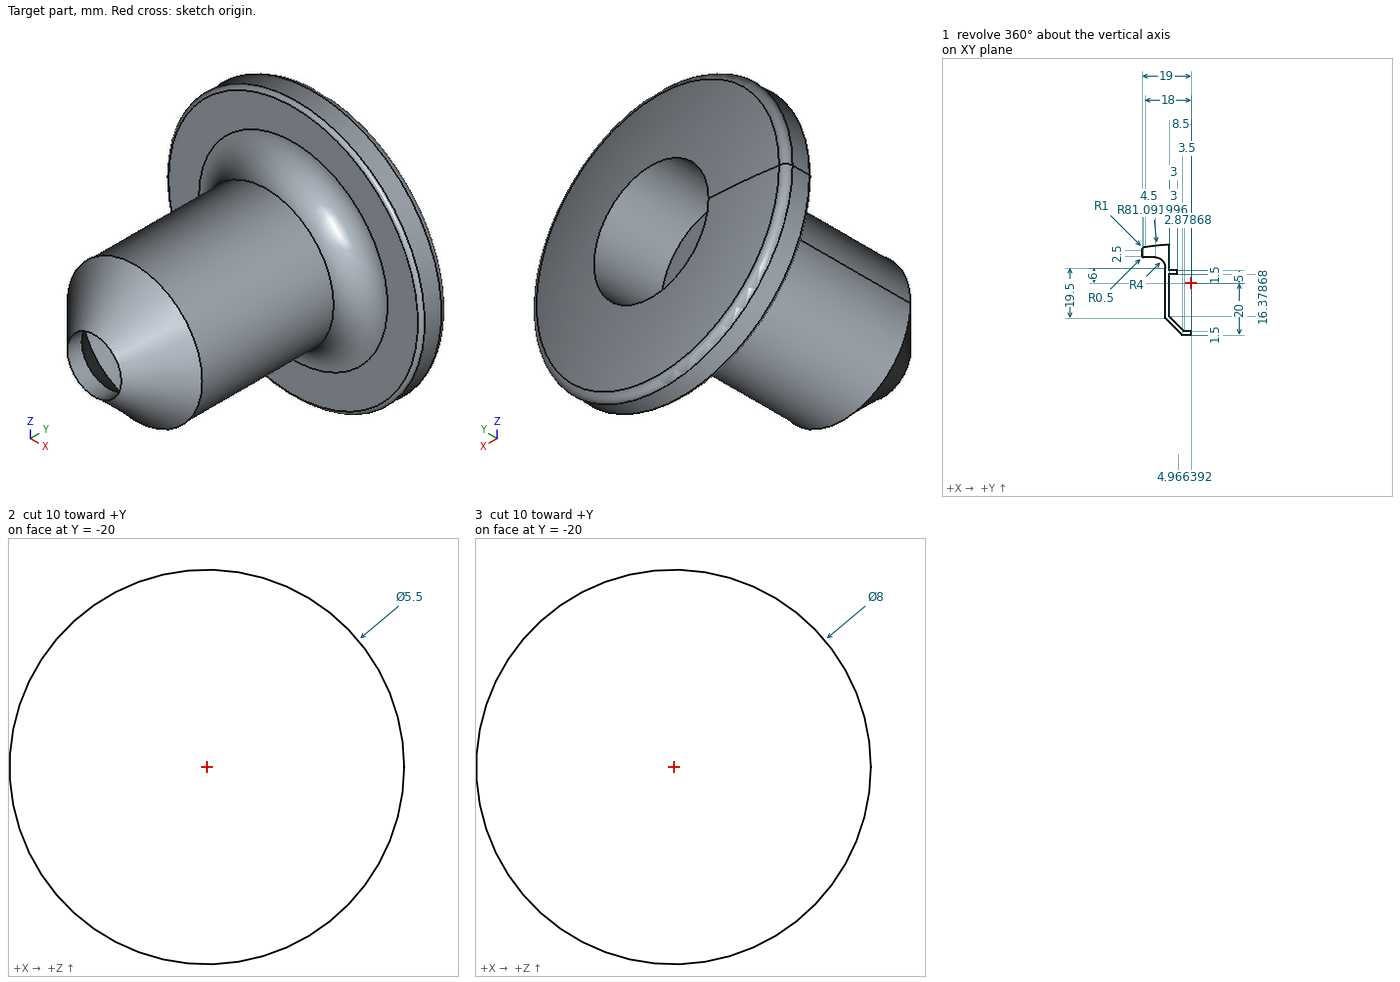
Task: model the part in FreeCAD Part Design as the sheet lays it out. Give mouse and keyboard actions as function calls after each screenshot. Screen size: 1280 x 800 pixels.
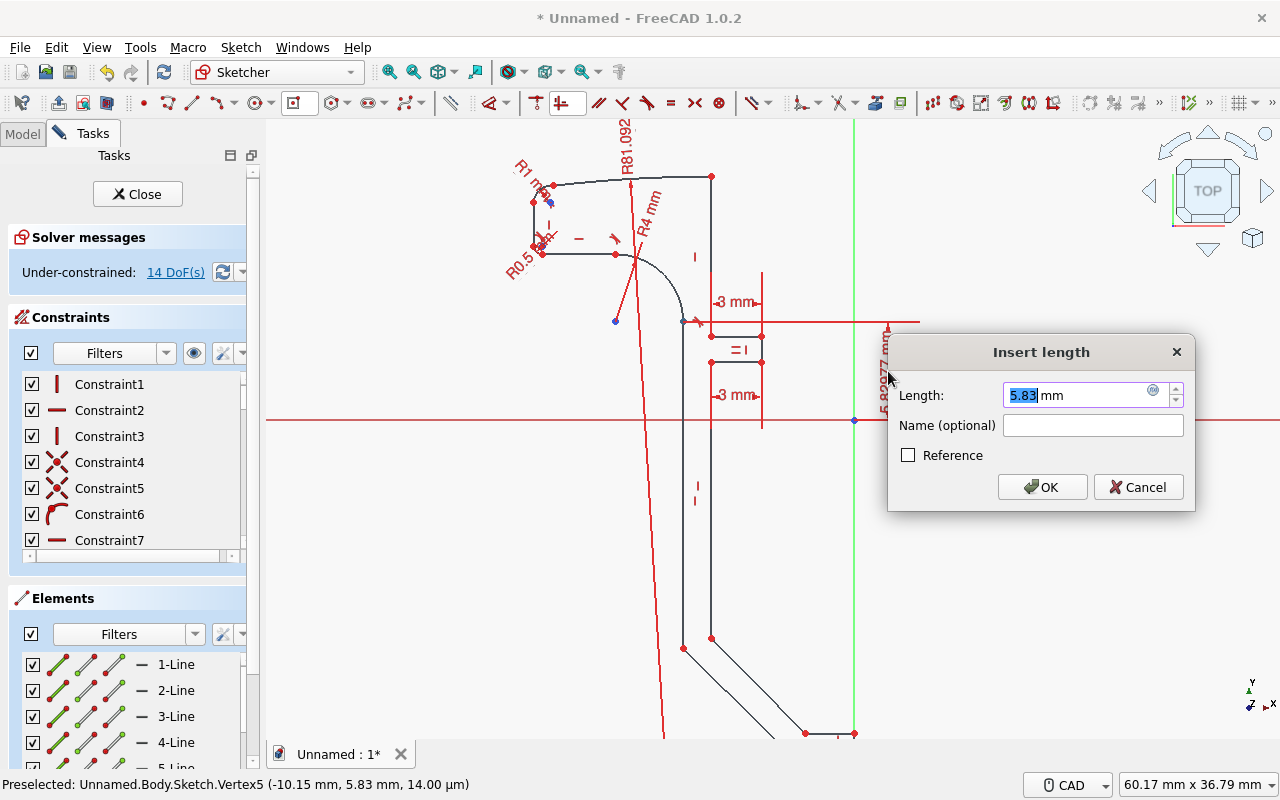
text(6)
key(Return)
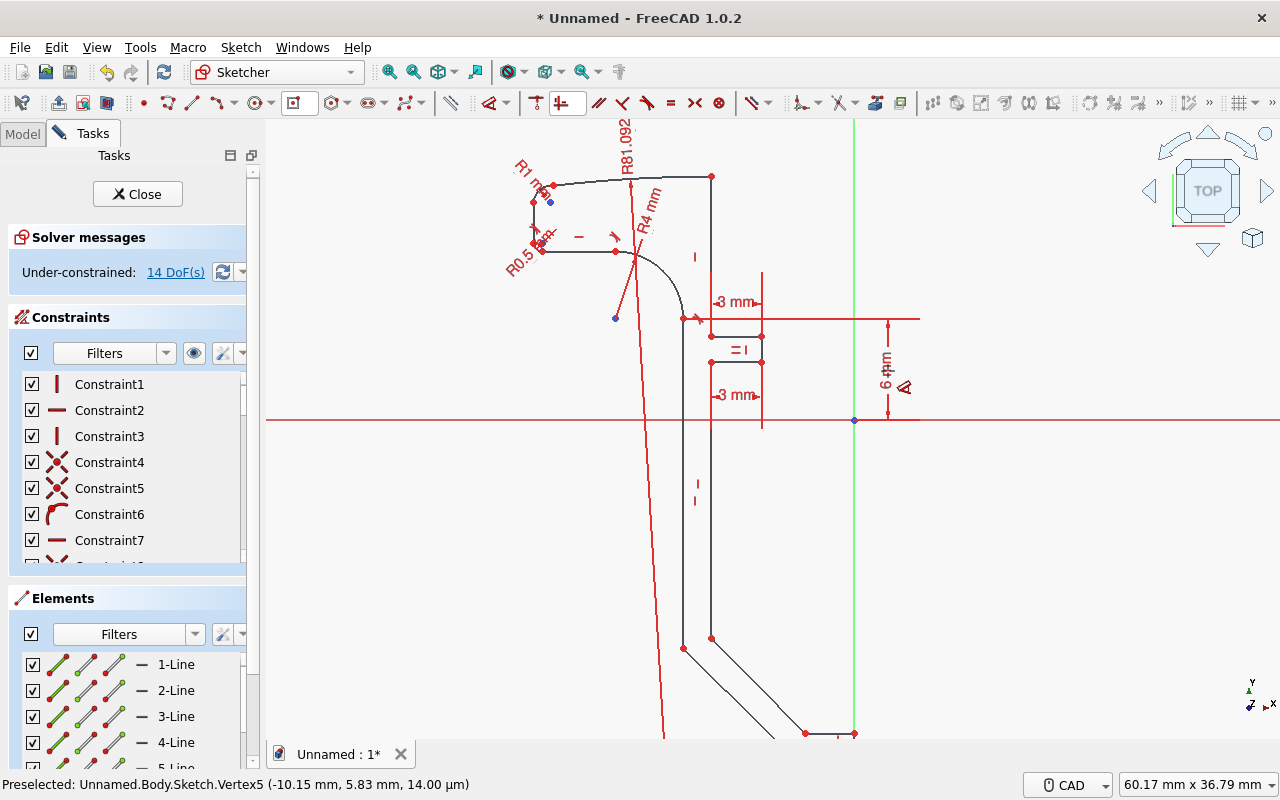
click(762, 337)
click(888, 398)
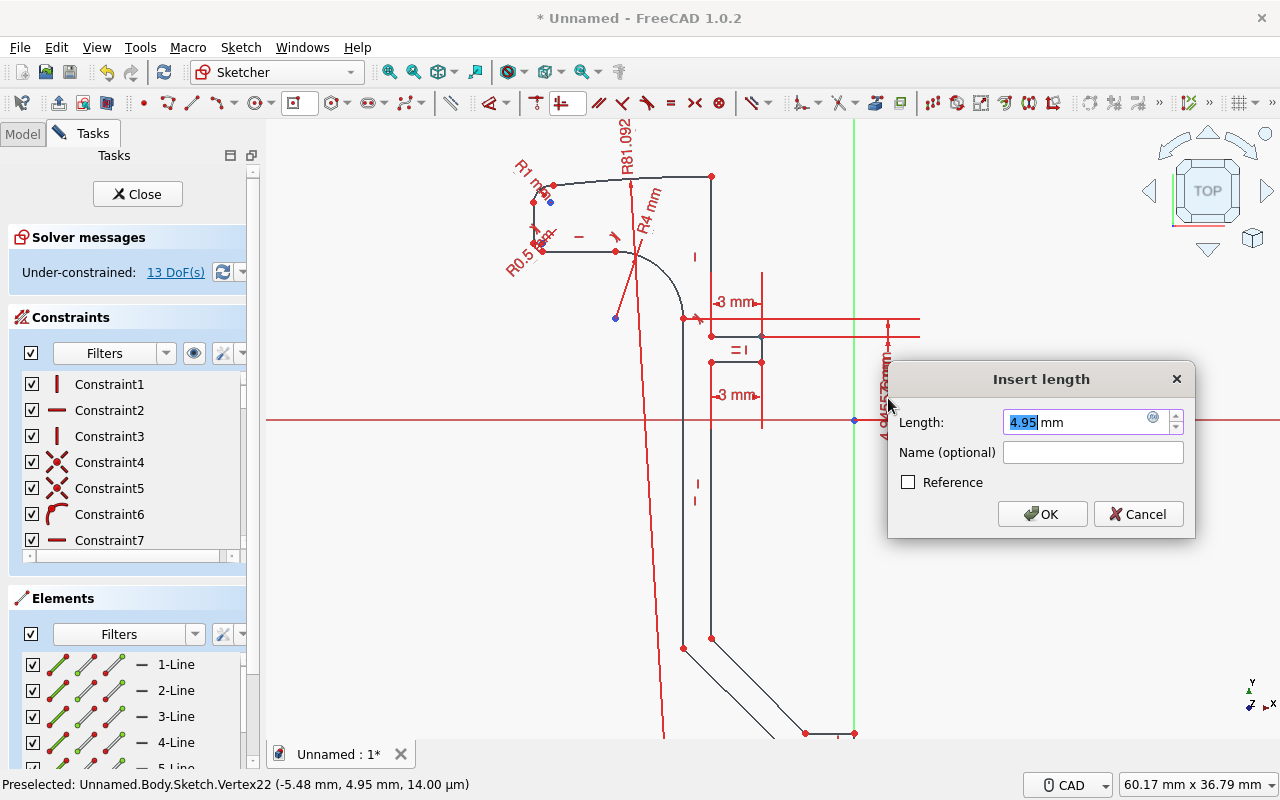
text(5)
key(Return)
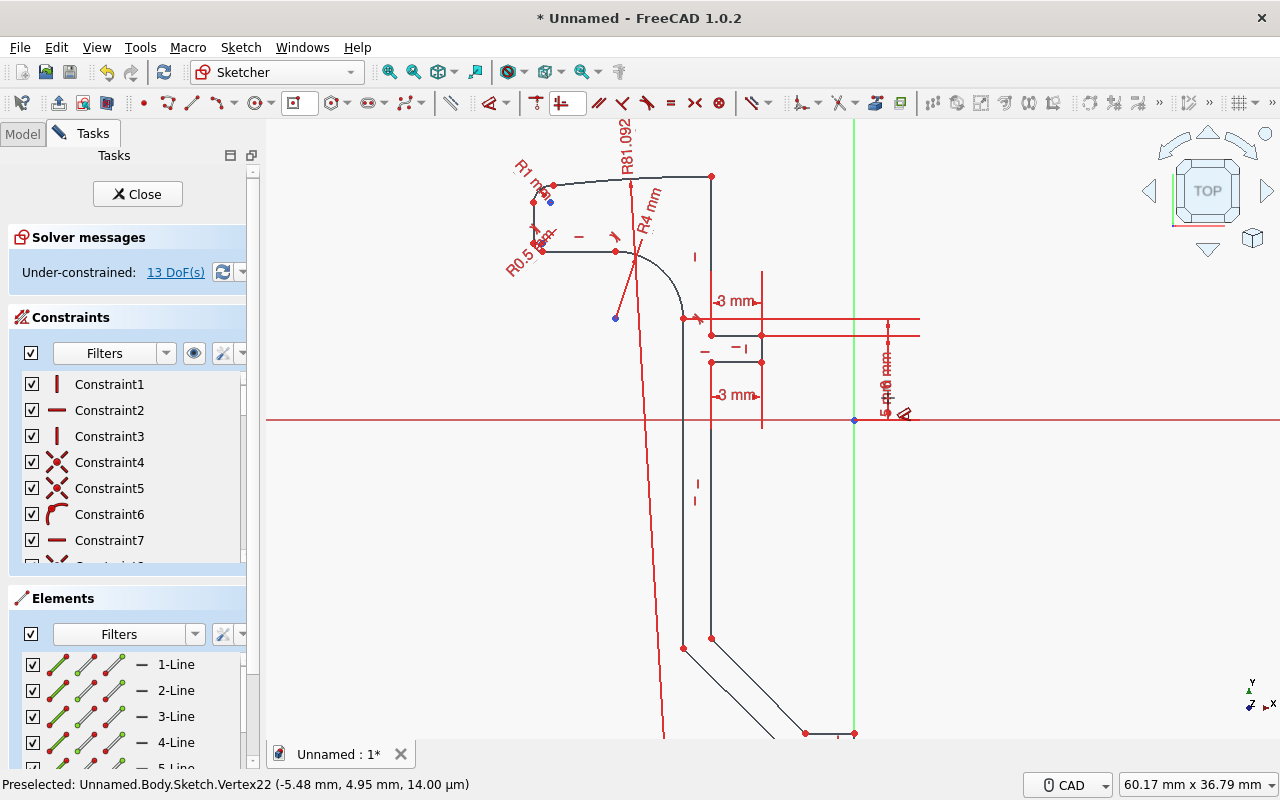
click(534, 215)
click(500, 223)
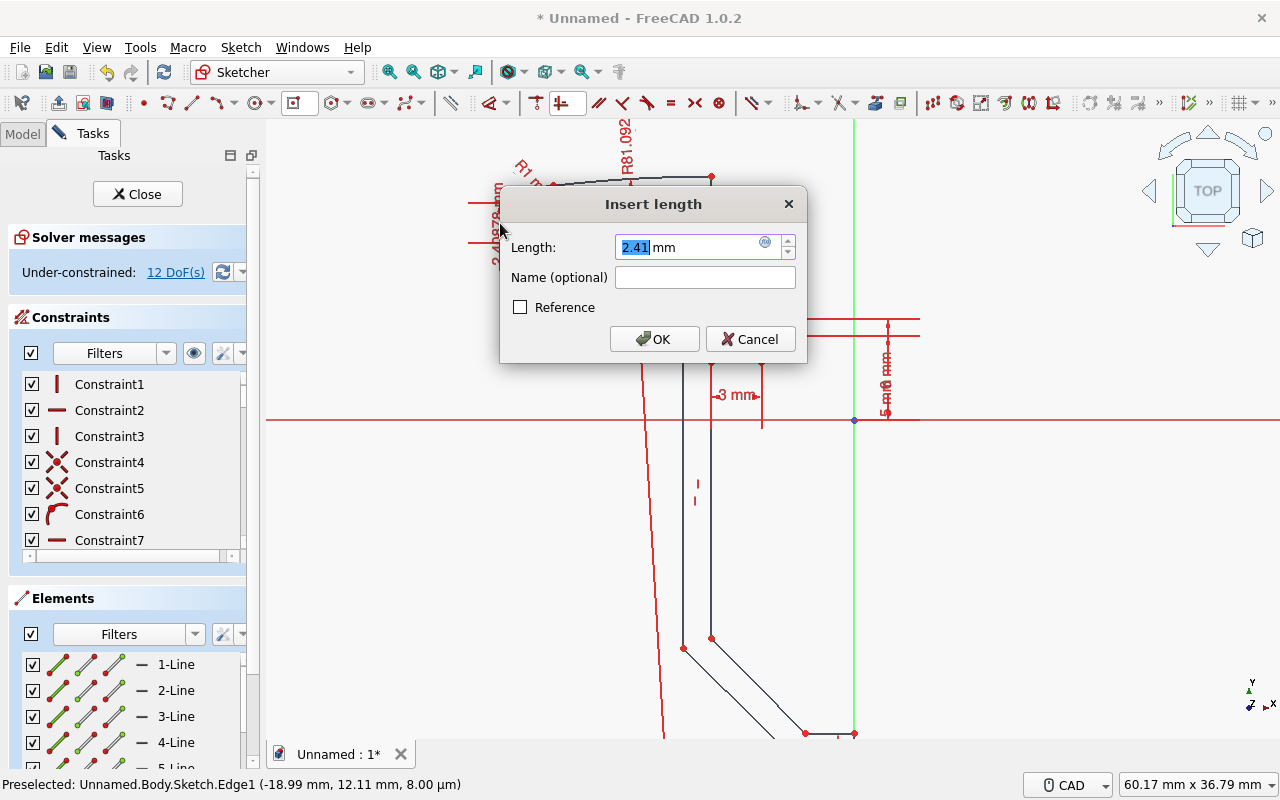
text(2.5)
key(Return)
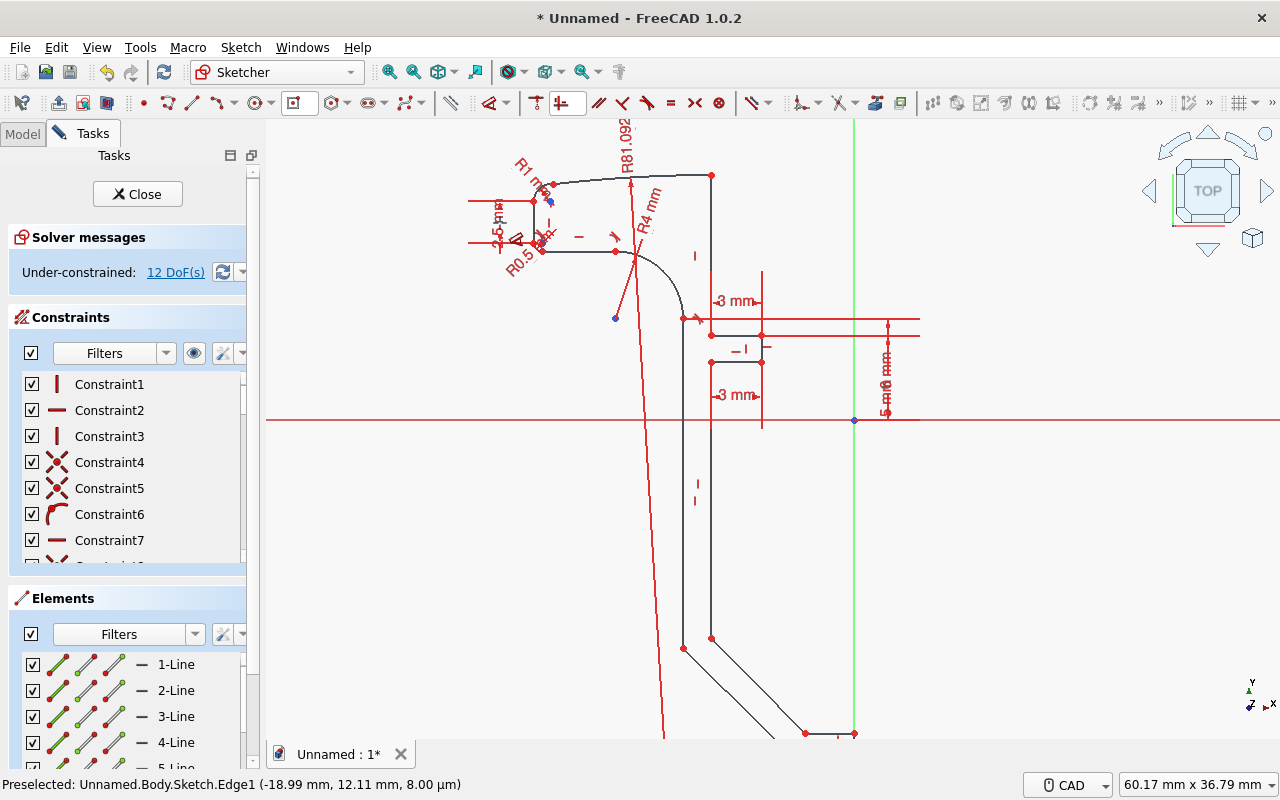
click(564, 252)
click(579, 218)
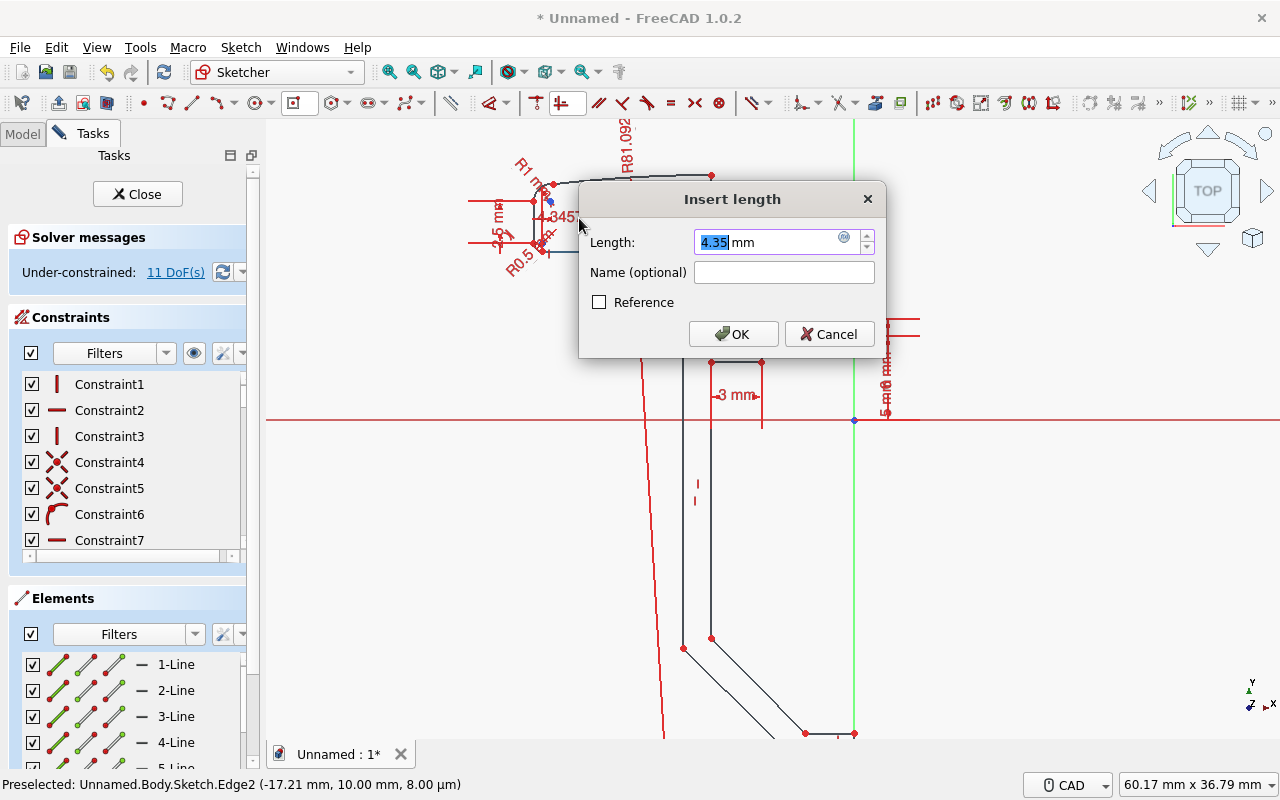
text(4.5)
key(Return)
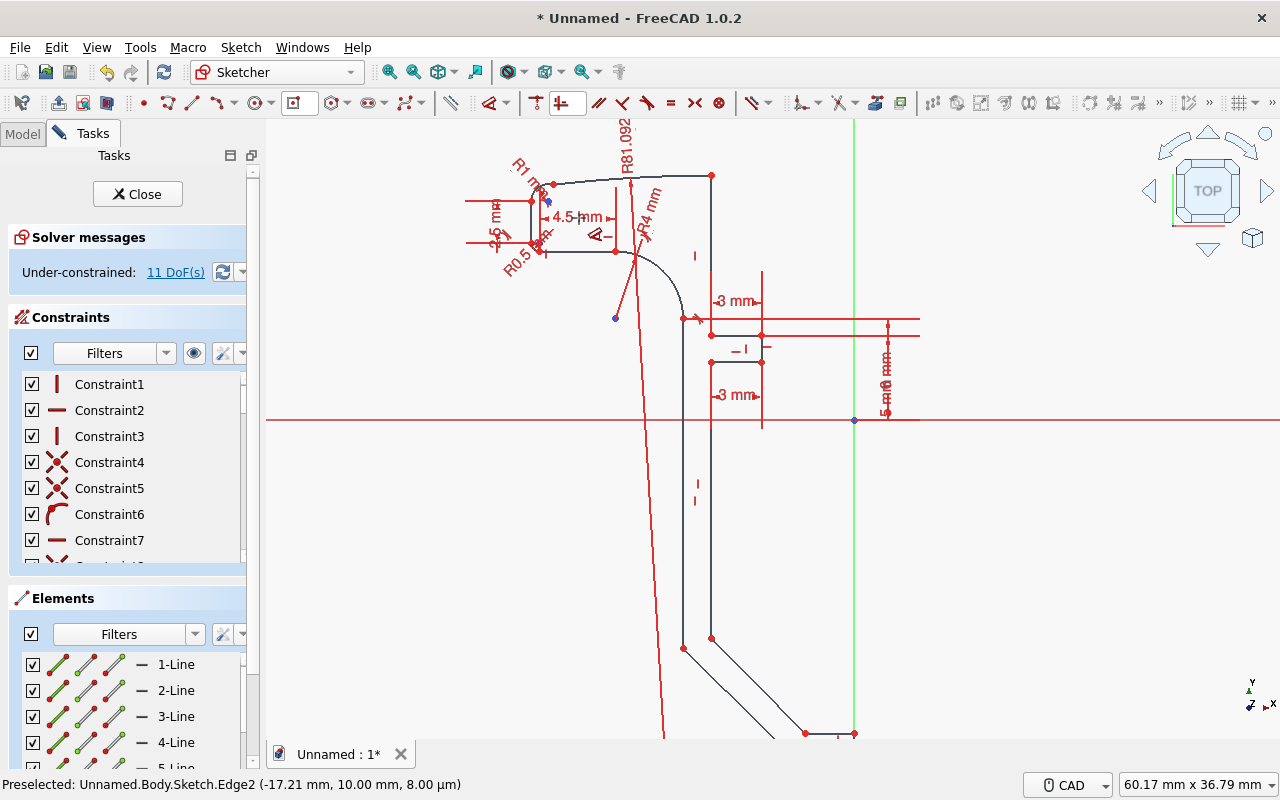
scroll(726, 361, down, 2)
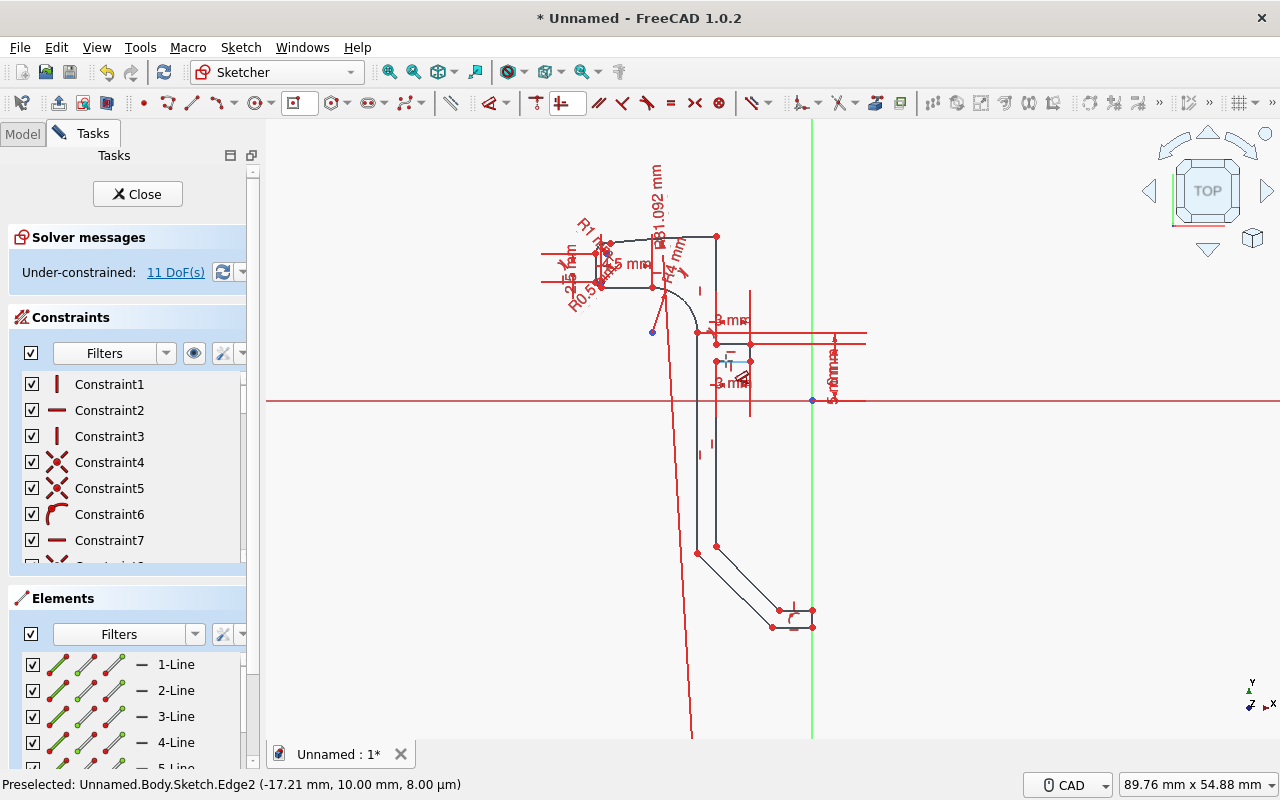
click(784, 628)
click(792, 662)